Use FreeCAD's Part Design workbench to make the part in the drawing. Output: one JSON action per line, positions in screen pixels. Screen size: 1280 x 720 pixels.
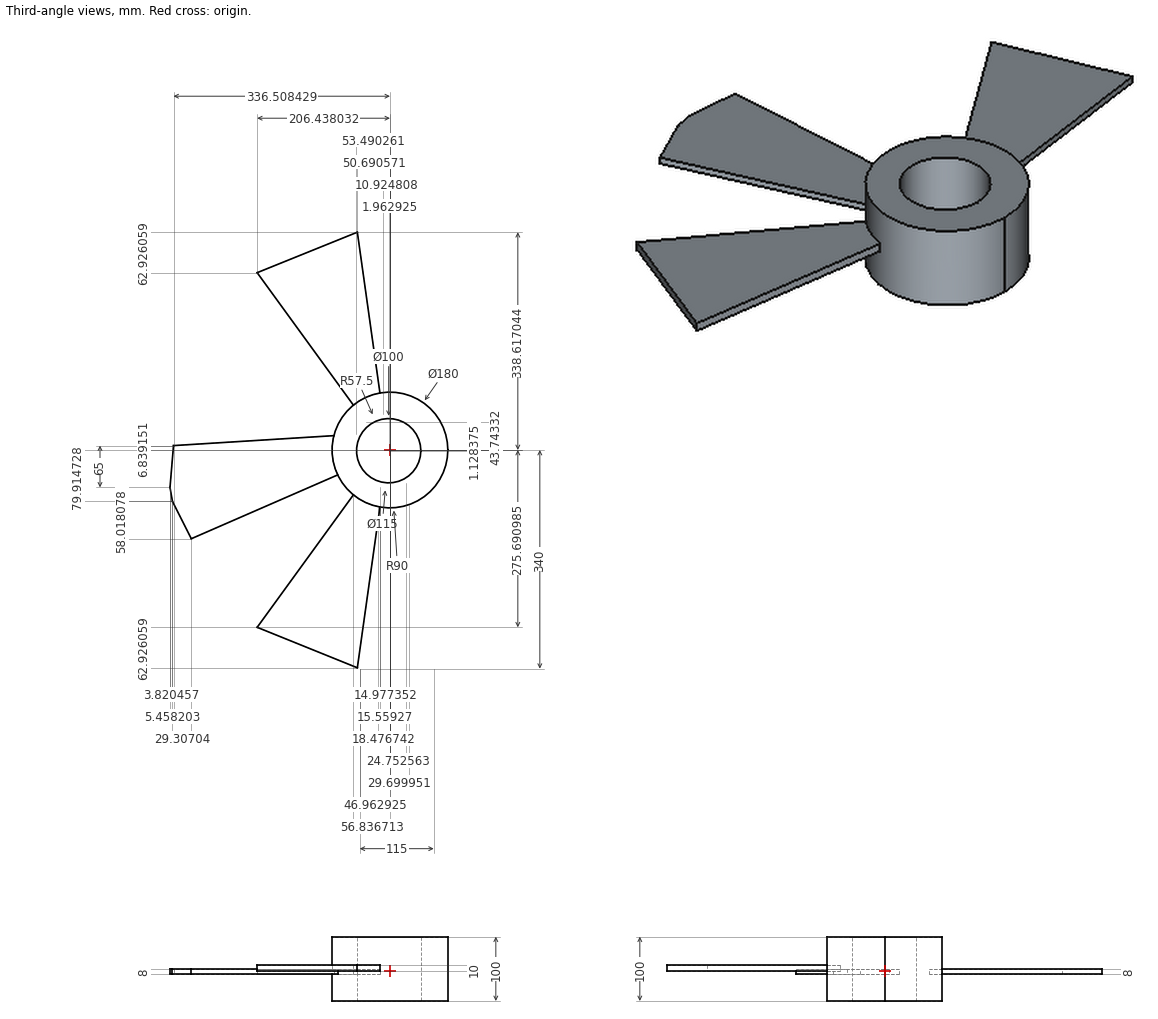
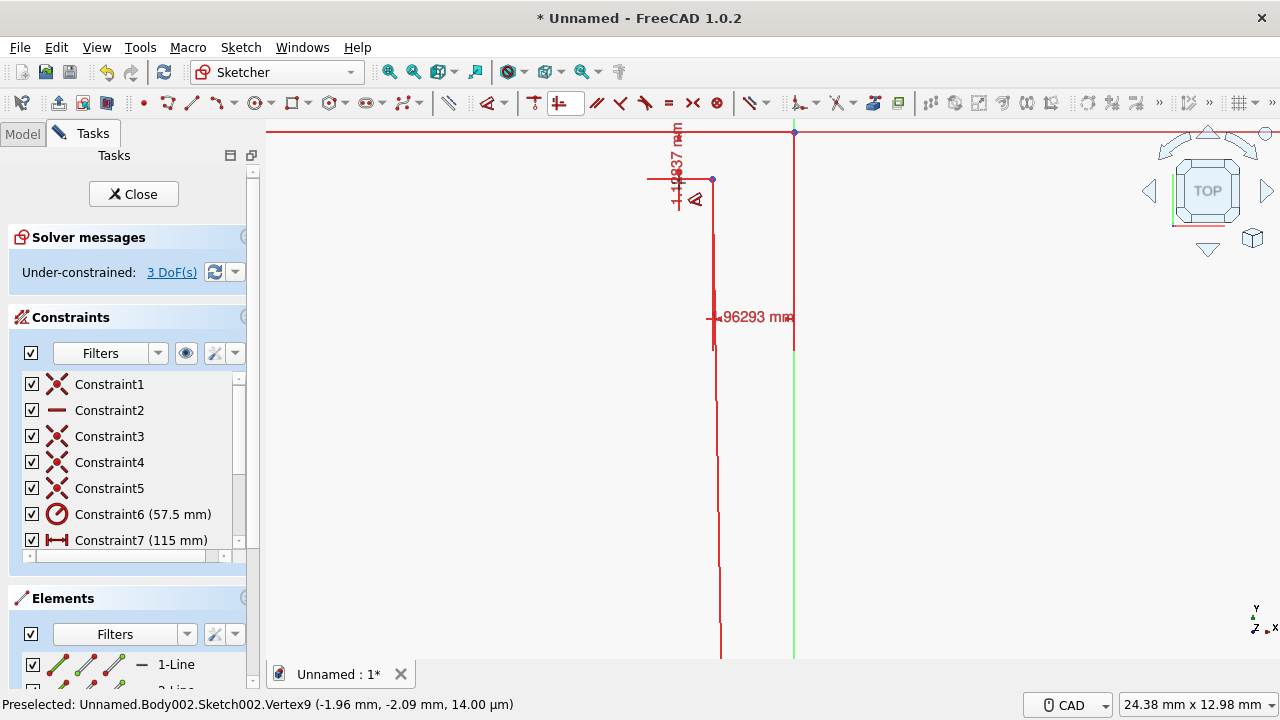
{"action": "scroll", "coordinate": [690, 198], "scroll_direction": "down", "scroll_amount": 18}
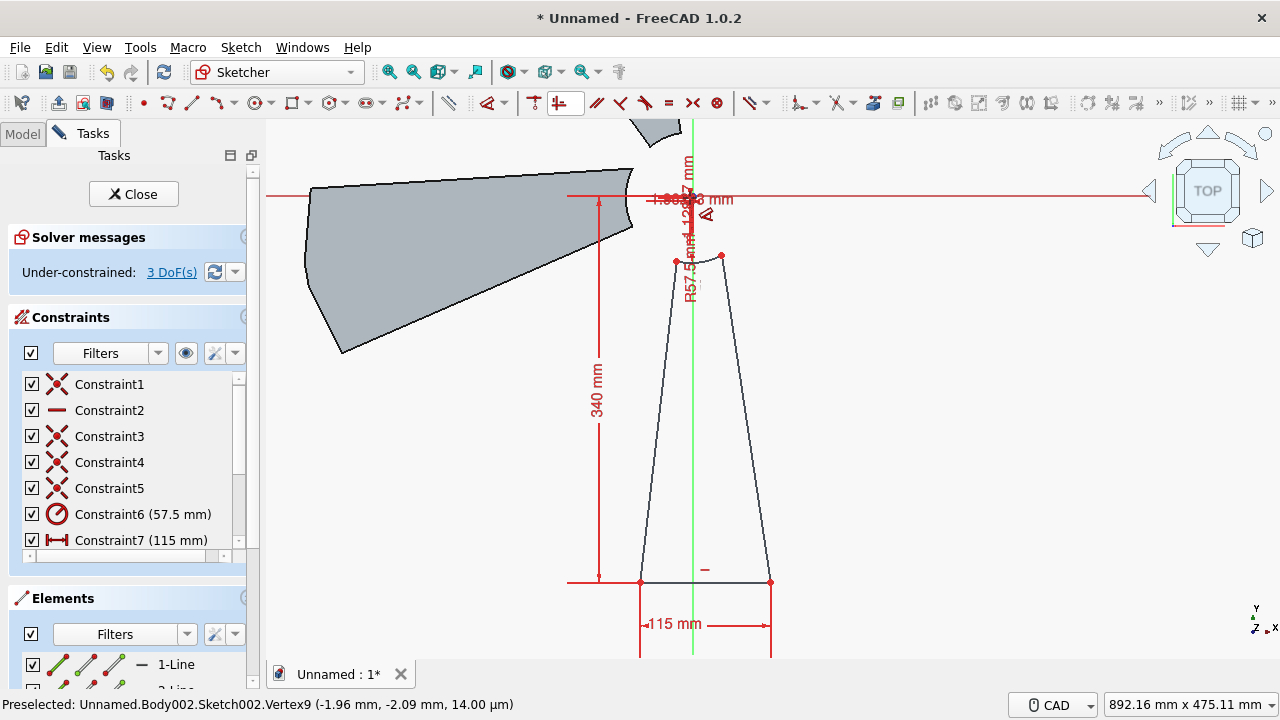
{"action": "scroll", "coordinate": [677, 261], "scroll_direction": "up", "scroll_amount": 5}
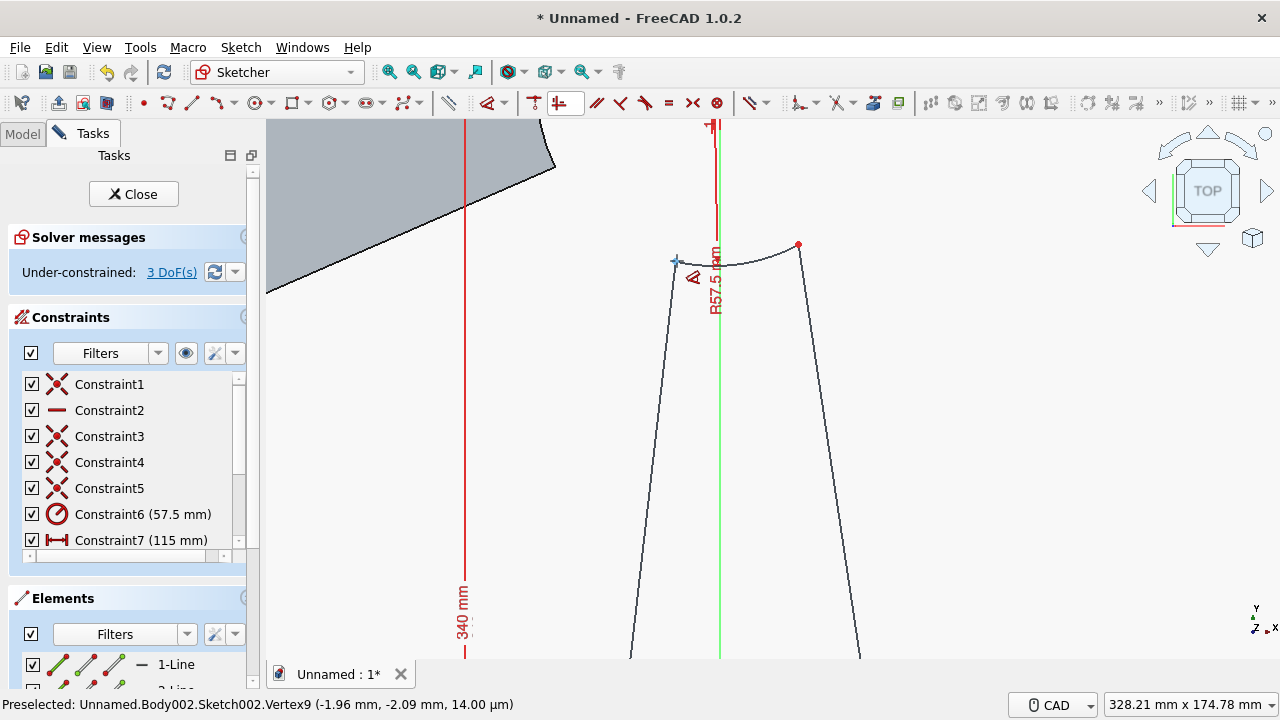
{"action": "left_click", "coordinate": [676, 262]}
{"action": "left_click", "coordinate": [698, 320]}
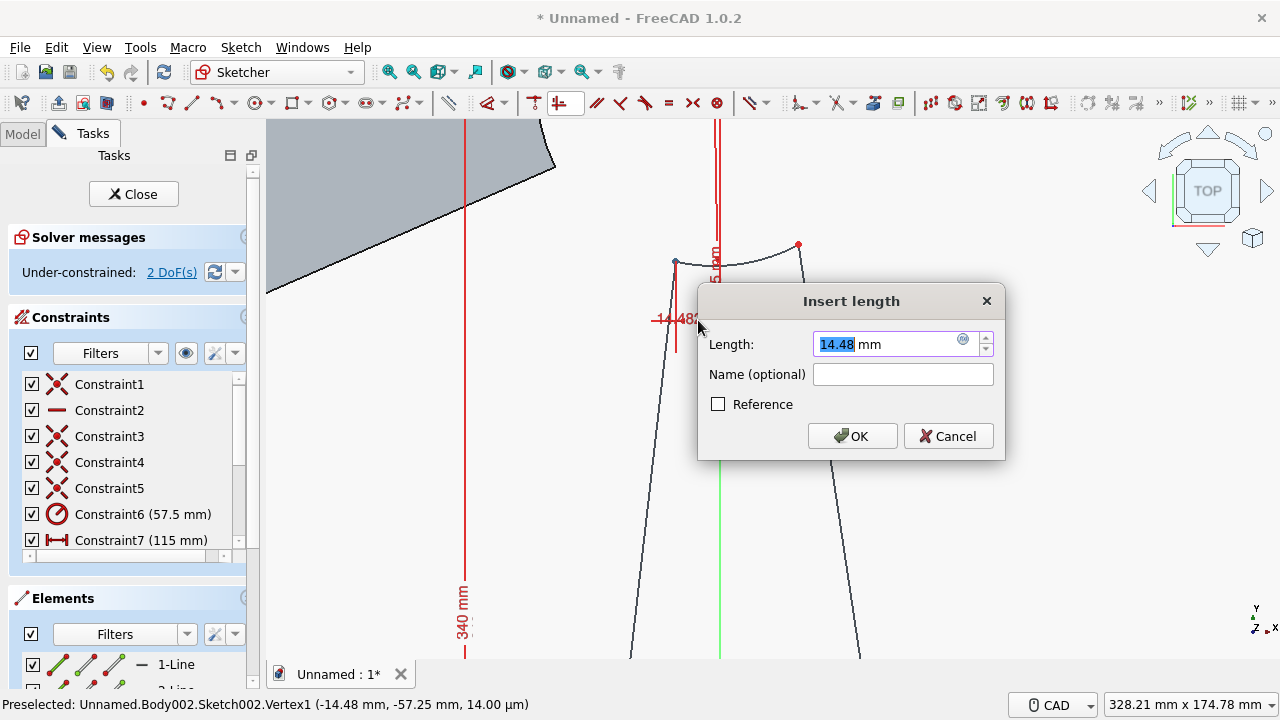
{"action": "type", "text": "14.977352"}
{"action": "key", "text": "Return"}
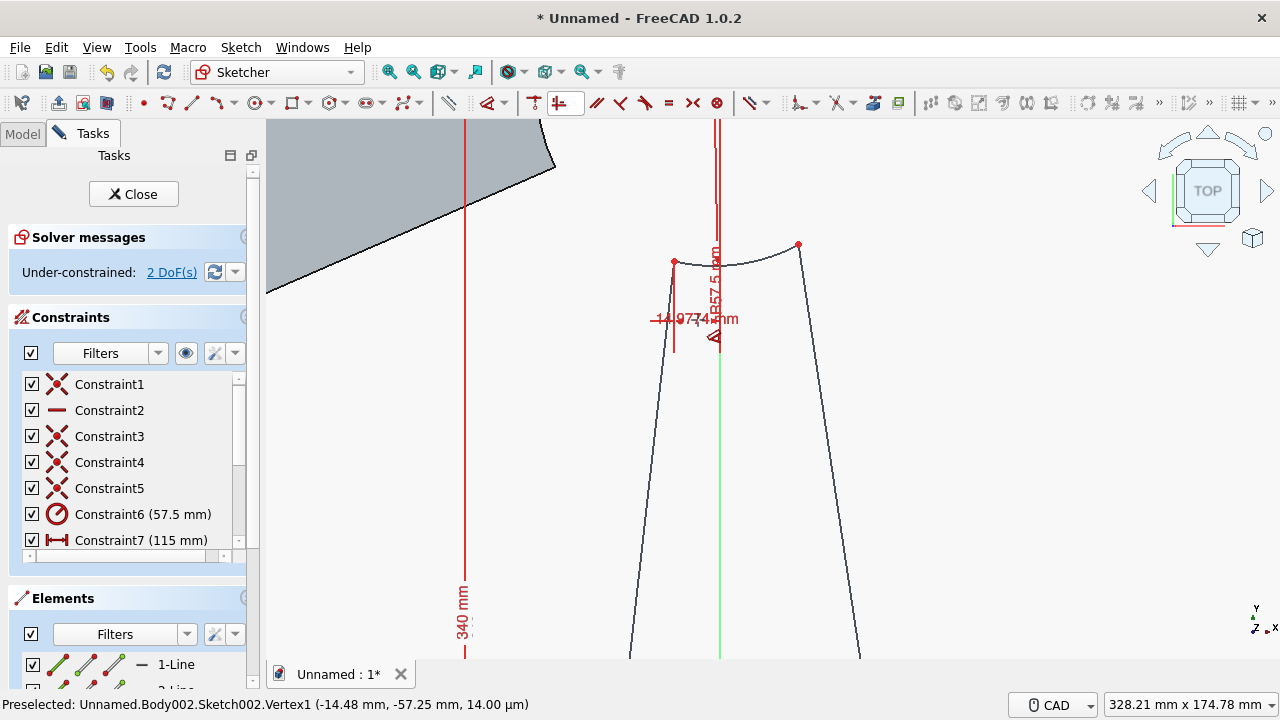
{"action": "scroll", "coordinate": [684, 294], "scroll_direction": "down", "scroll_amount": 6}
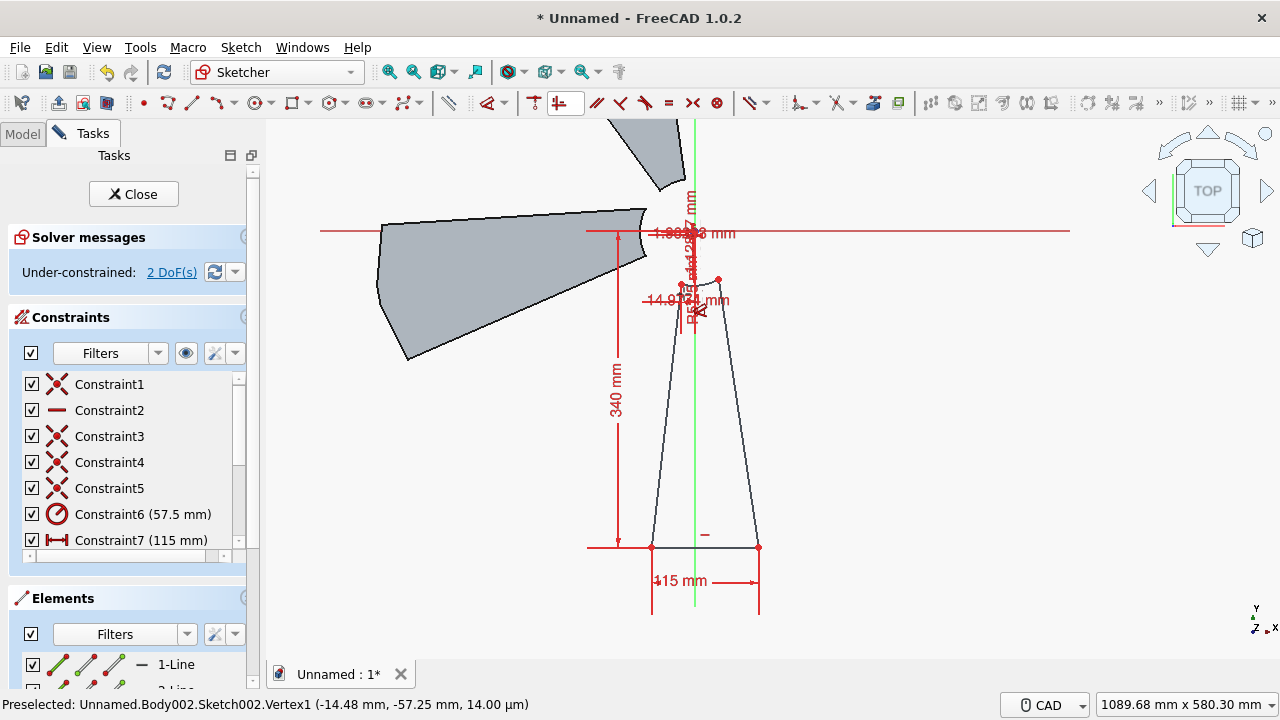
{"action": "left_click", "coordinate": [652, 548]}
{"action": "left_click", "coordinate": [674, 197]}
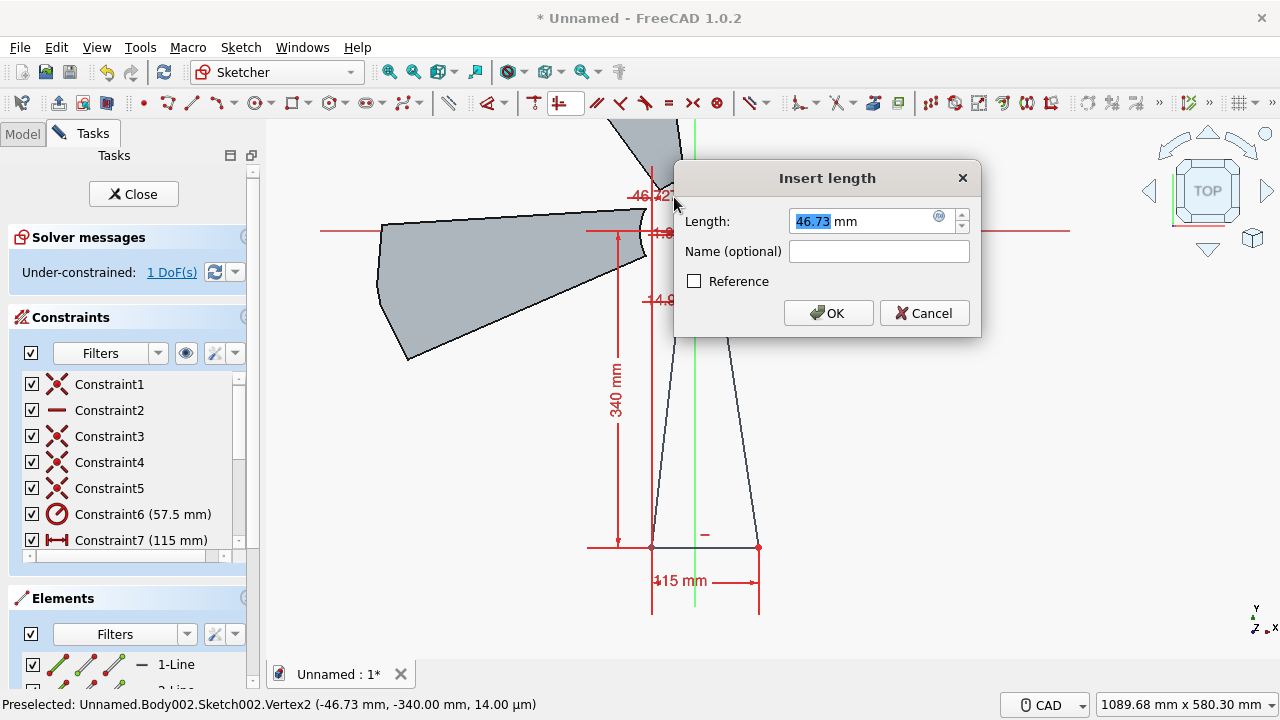
{"action": "type", "text": "46.962925"}
{"action": "key", "text": "Return"}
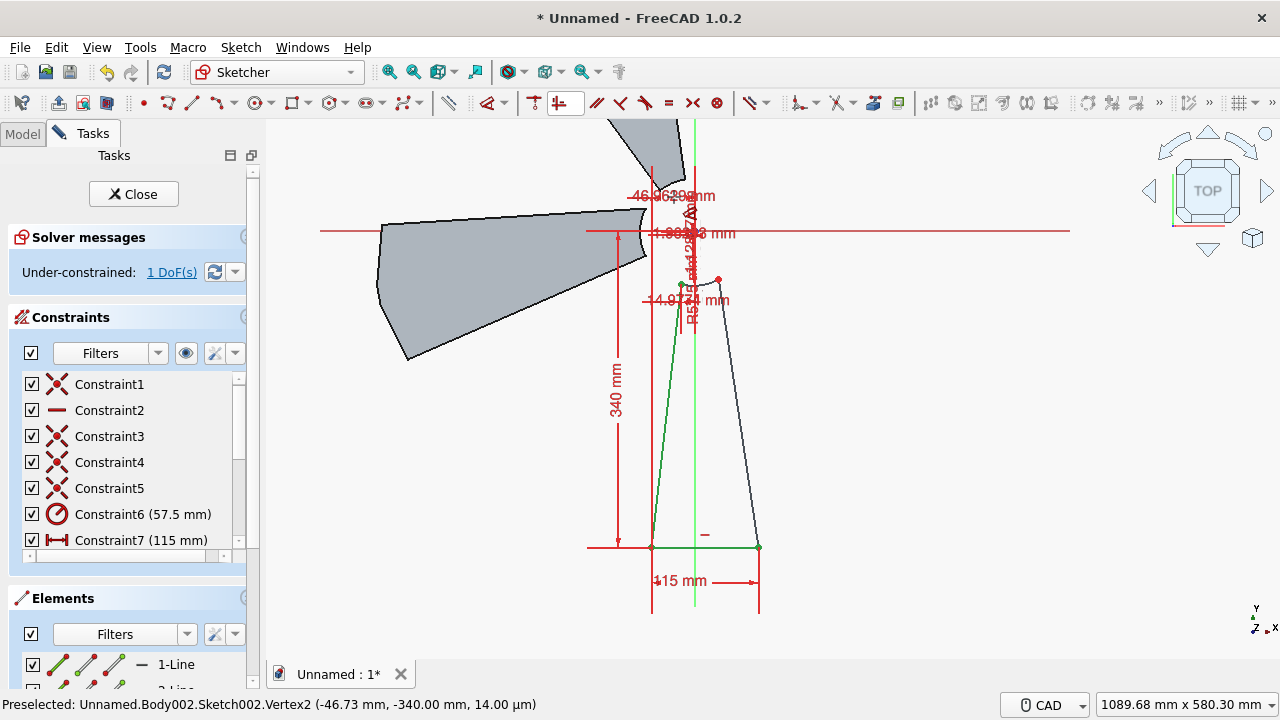
{"action": "scroll", "coordinate": [719, 279], "scroll_direction": "up", "scroll_amount": 3}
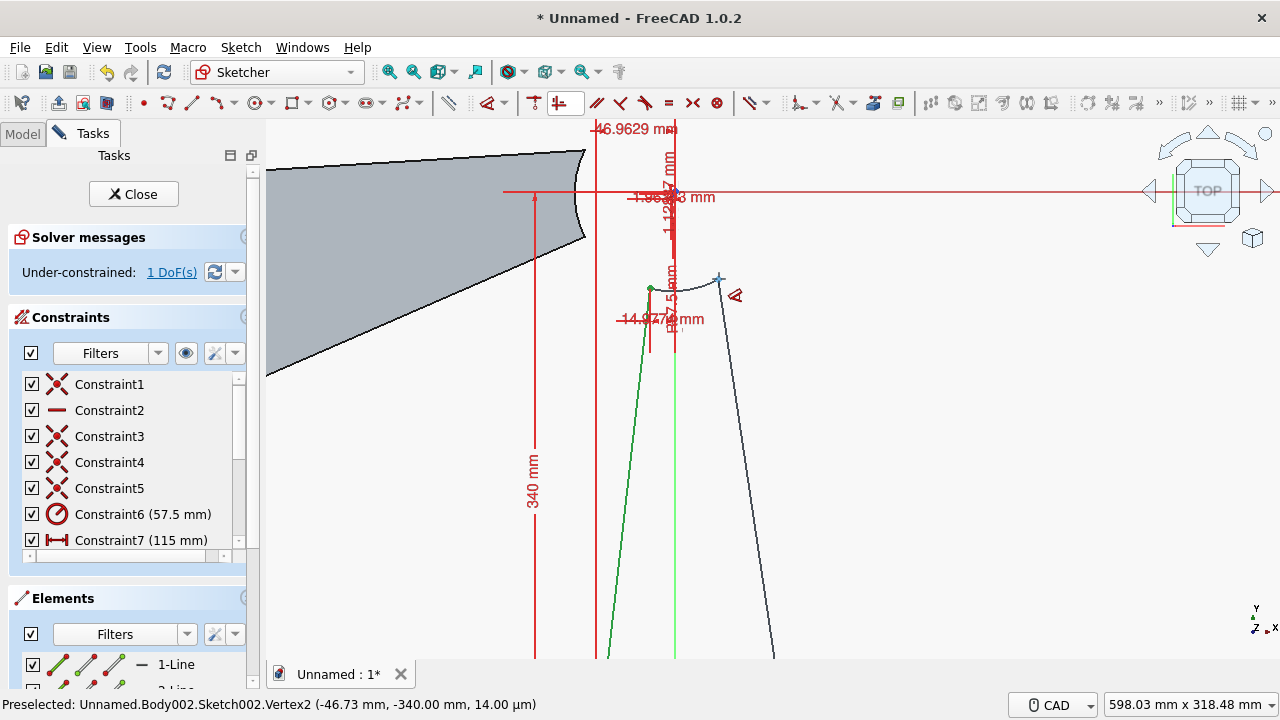
{"action": "left_click", "coordinate": [718, 279]}
{"action": "left_click", "coordinate": [697, 158]}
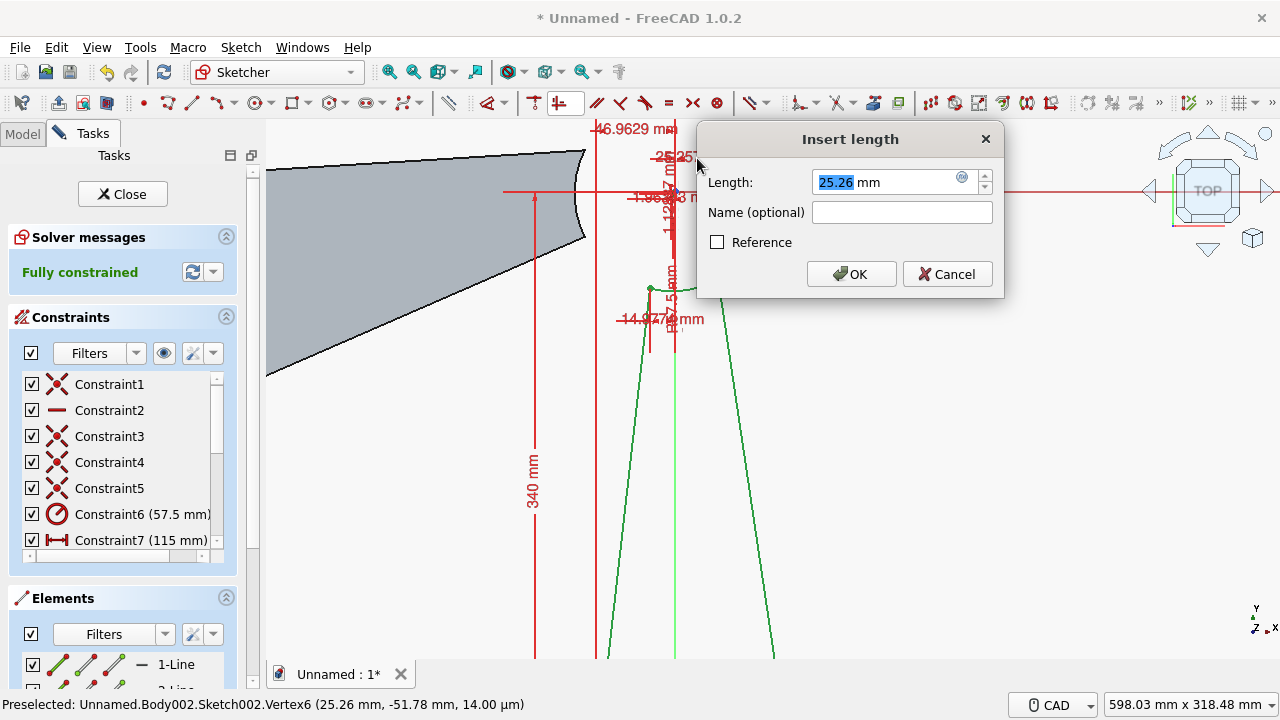
{"action": "type", "text": "24.752563"}
{"action": "key", "text": "Return"}
{"action": "key", "text": "Escape"}